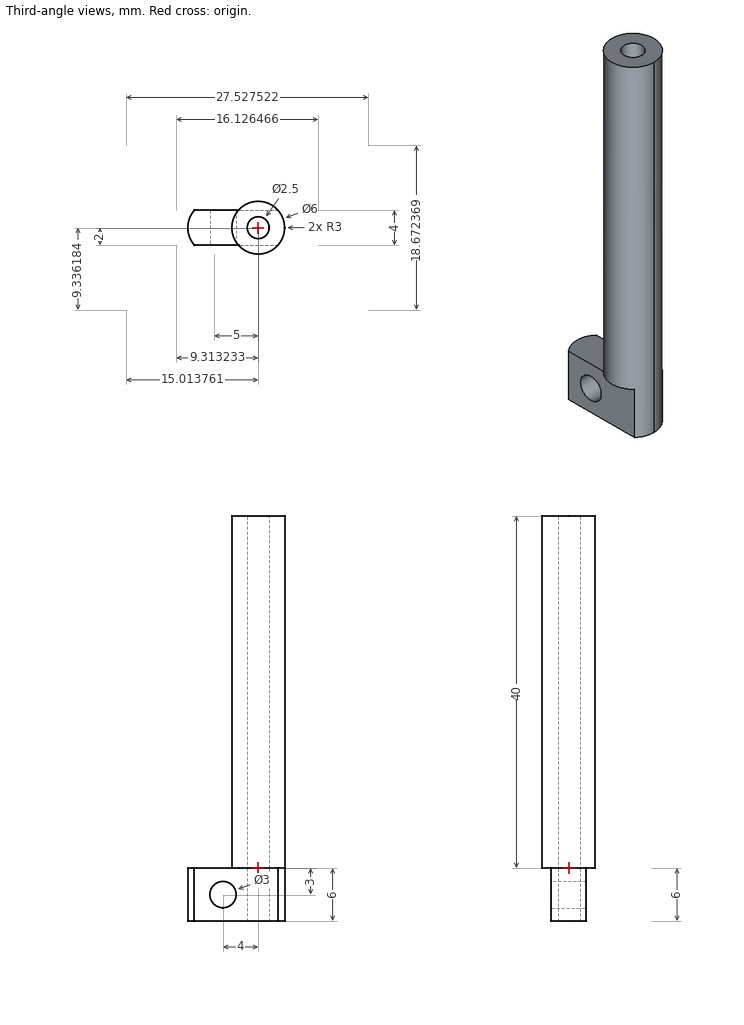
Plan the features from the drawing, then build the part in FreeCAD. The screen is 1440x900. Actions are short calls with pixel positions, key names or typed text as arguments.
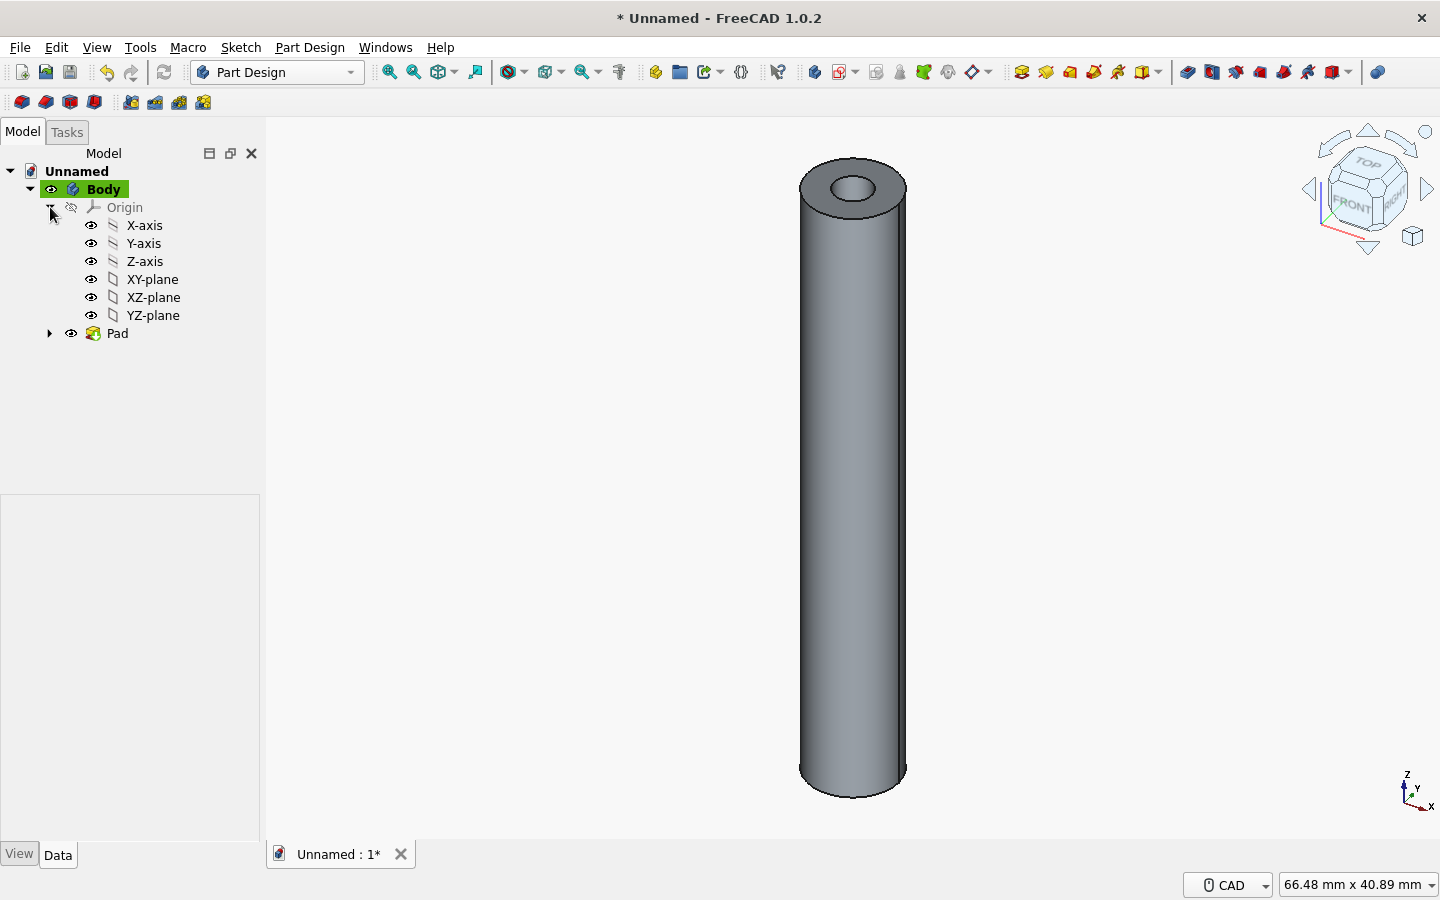
click(136, 279)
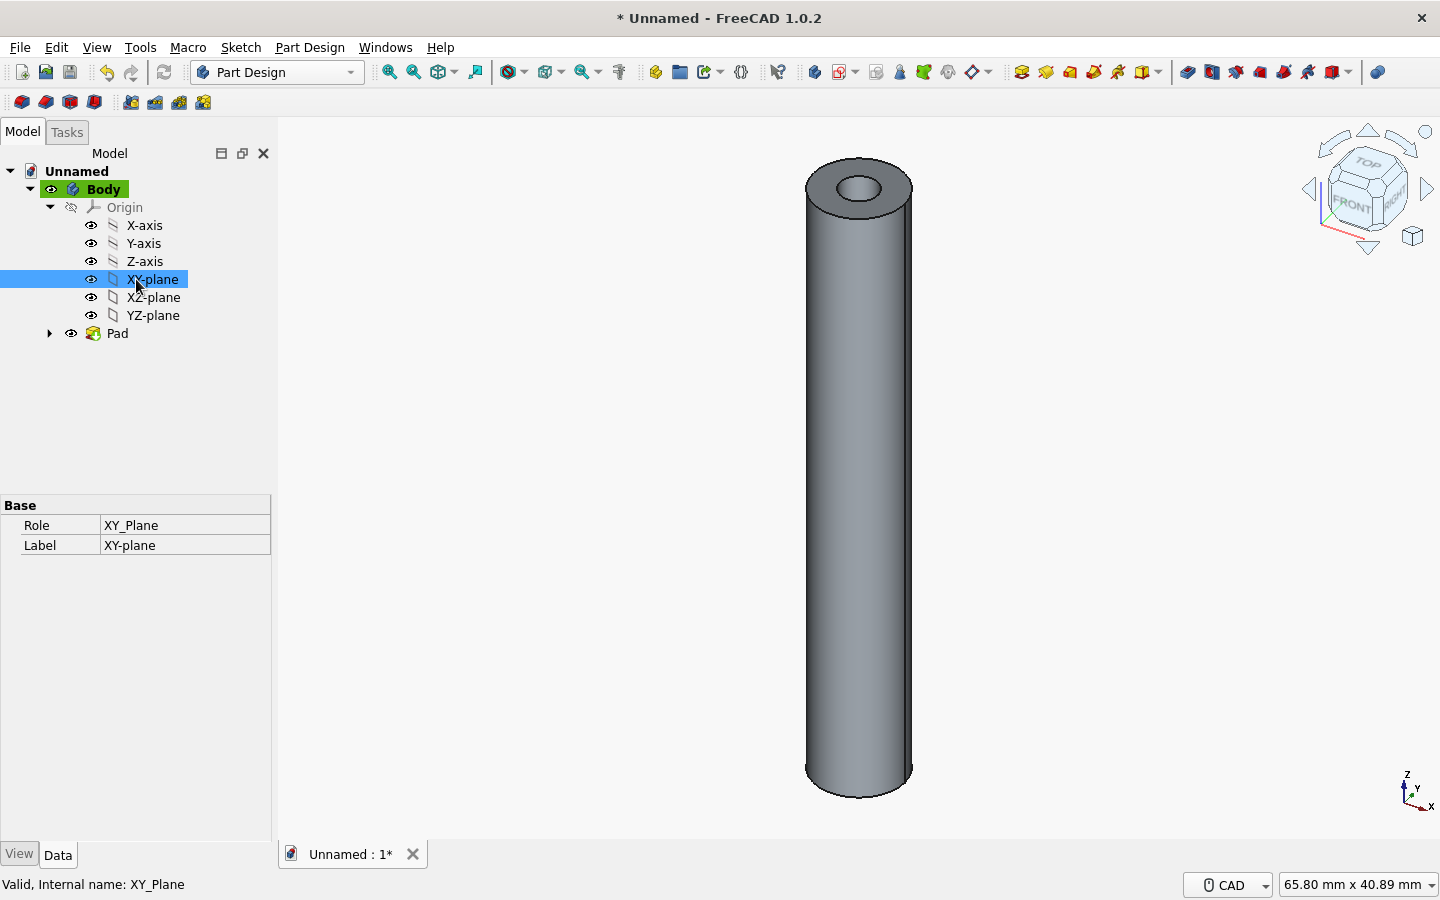
click(972, 72)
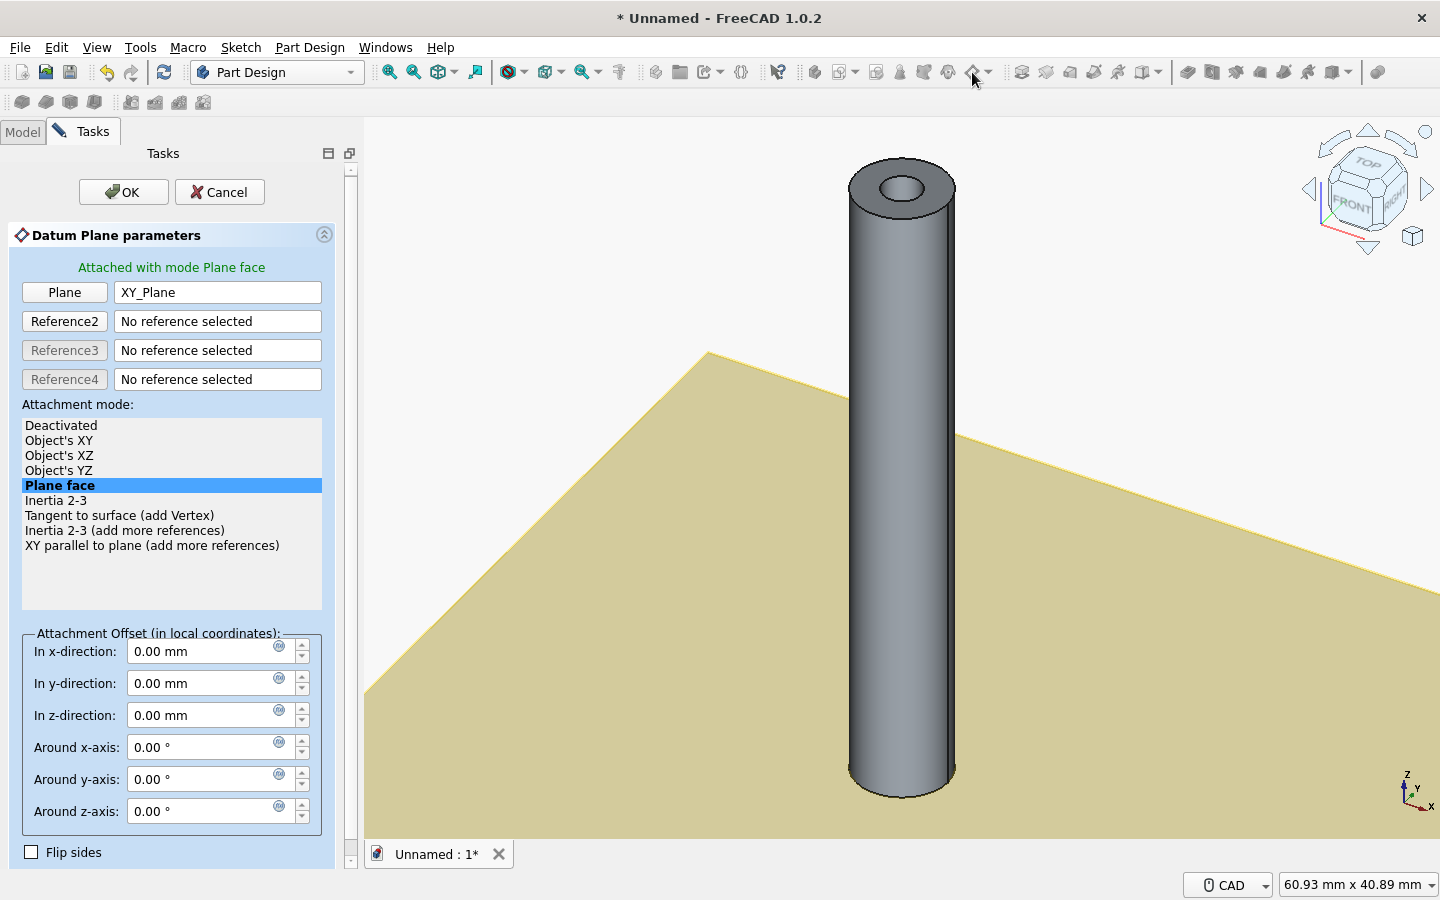
triple_click(210, 715)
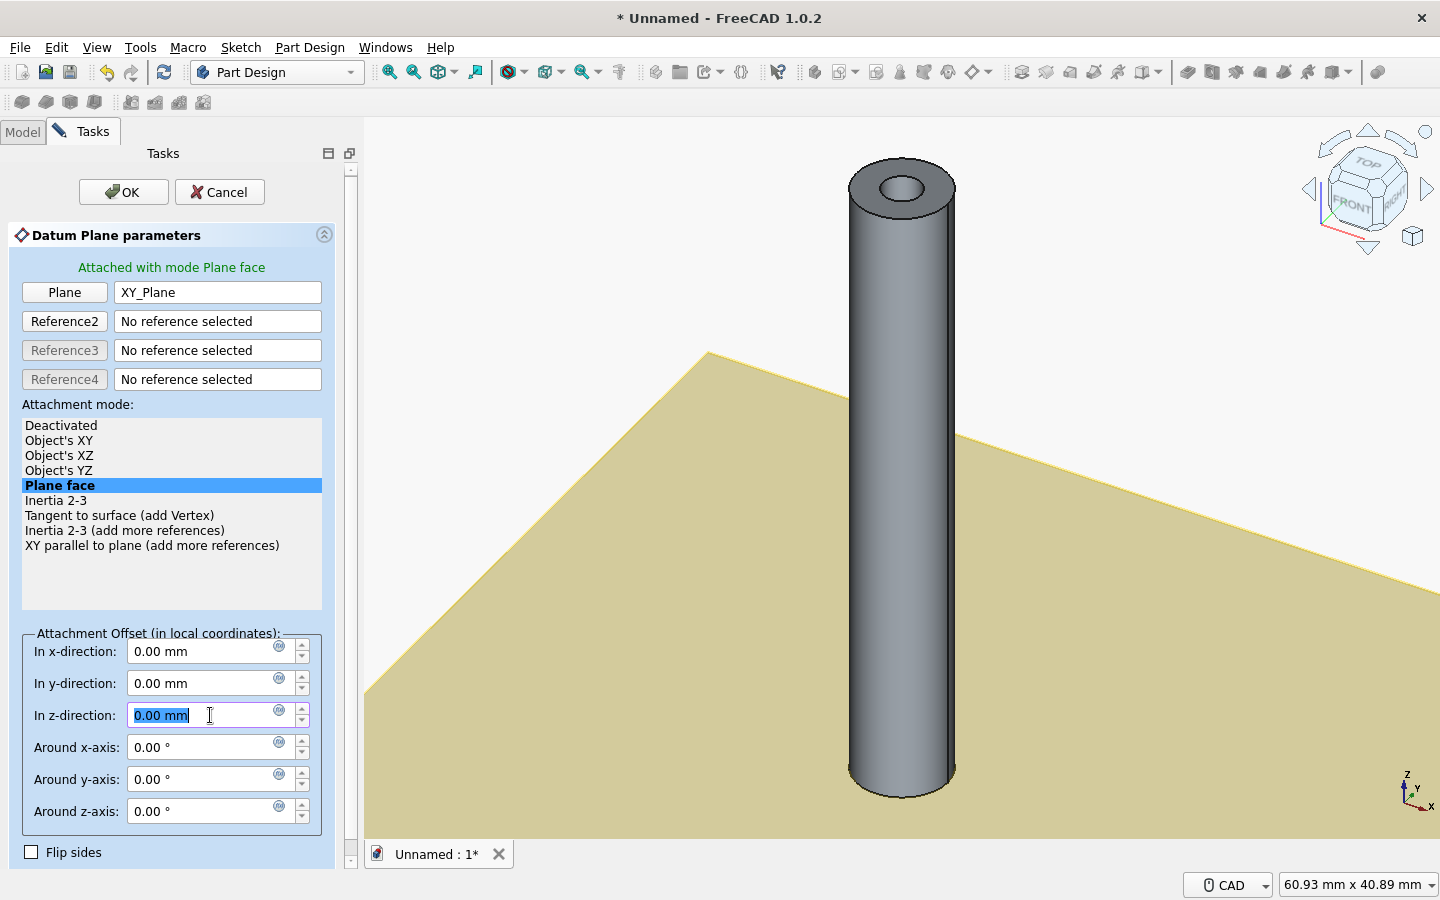
text(-6)
key(Tab)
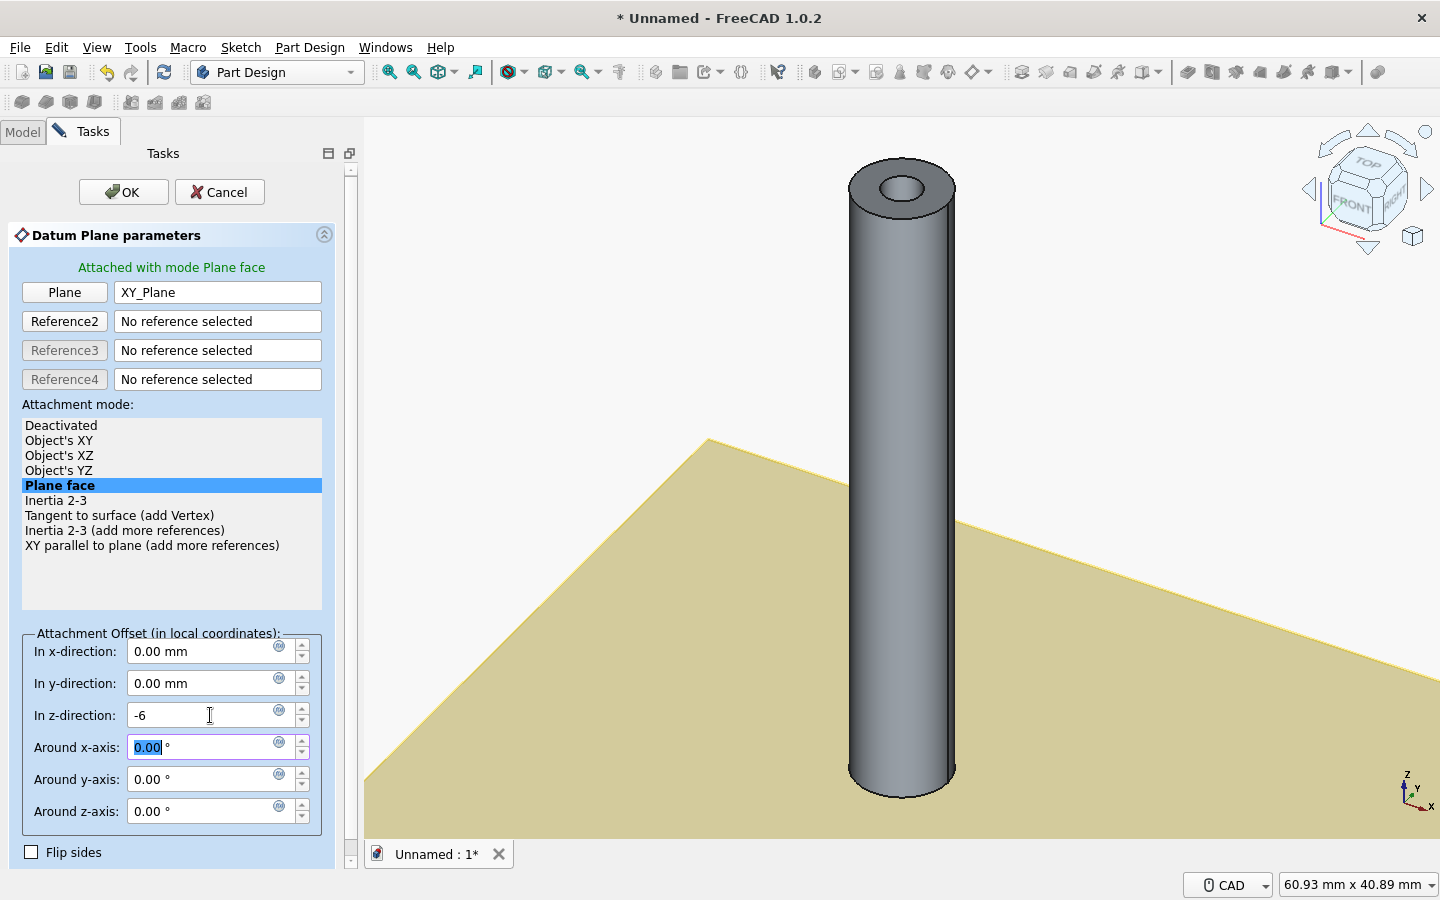
click(124, 192)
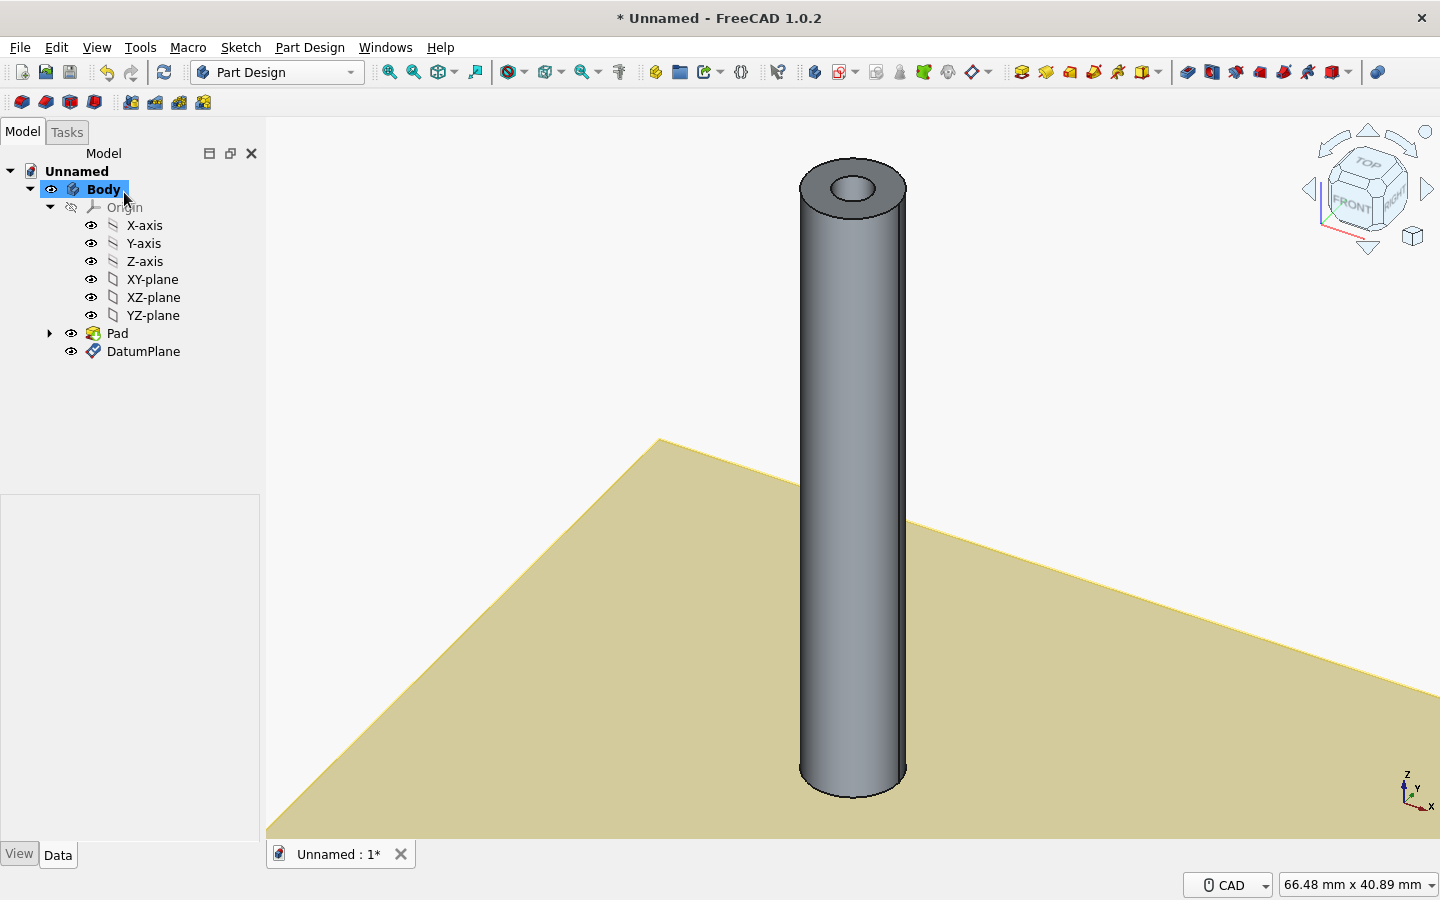
click(116, 351)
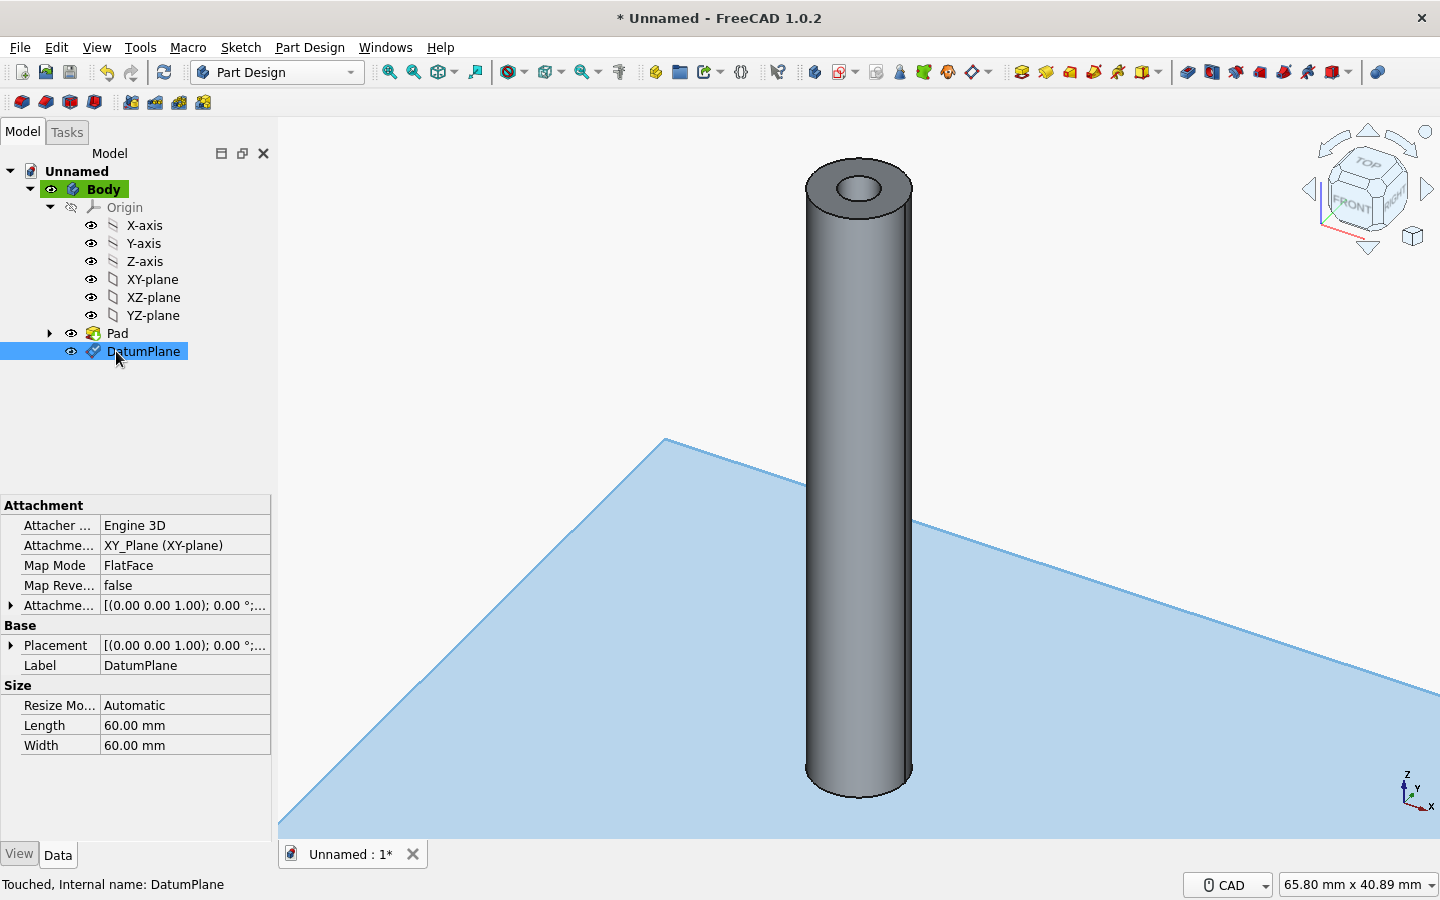
click(840, 72)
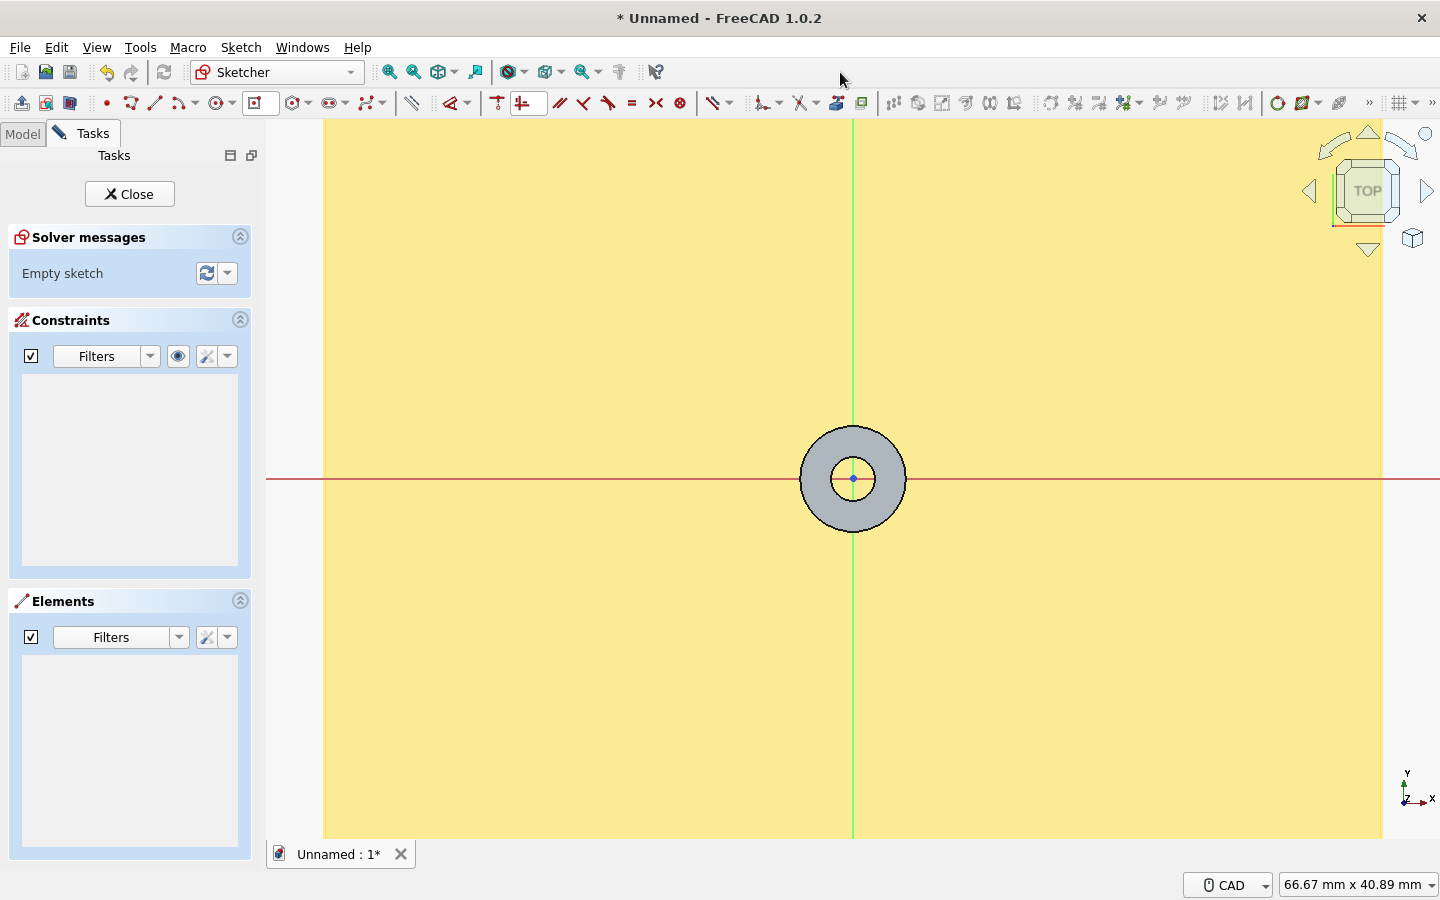
click(70, 104)